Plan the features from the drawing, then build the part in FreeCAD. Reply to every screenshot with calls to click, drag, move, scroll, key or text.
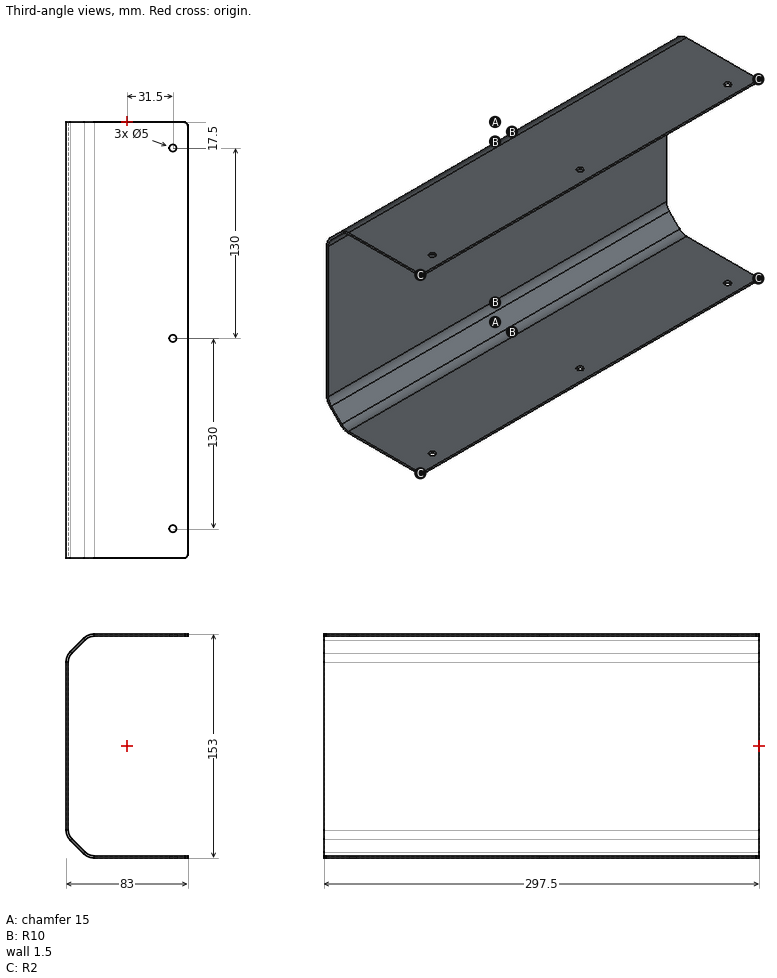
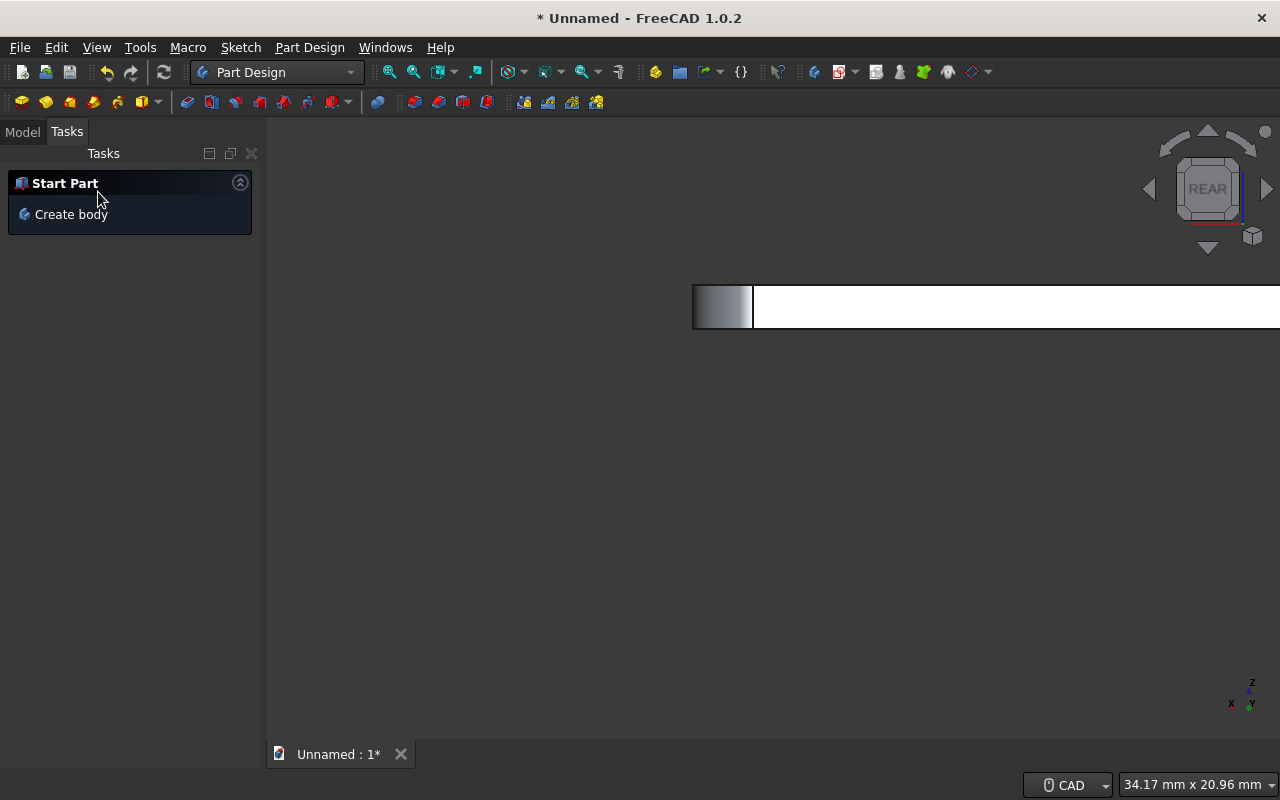
key(0)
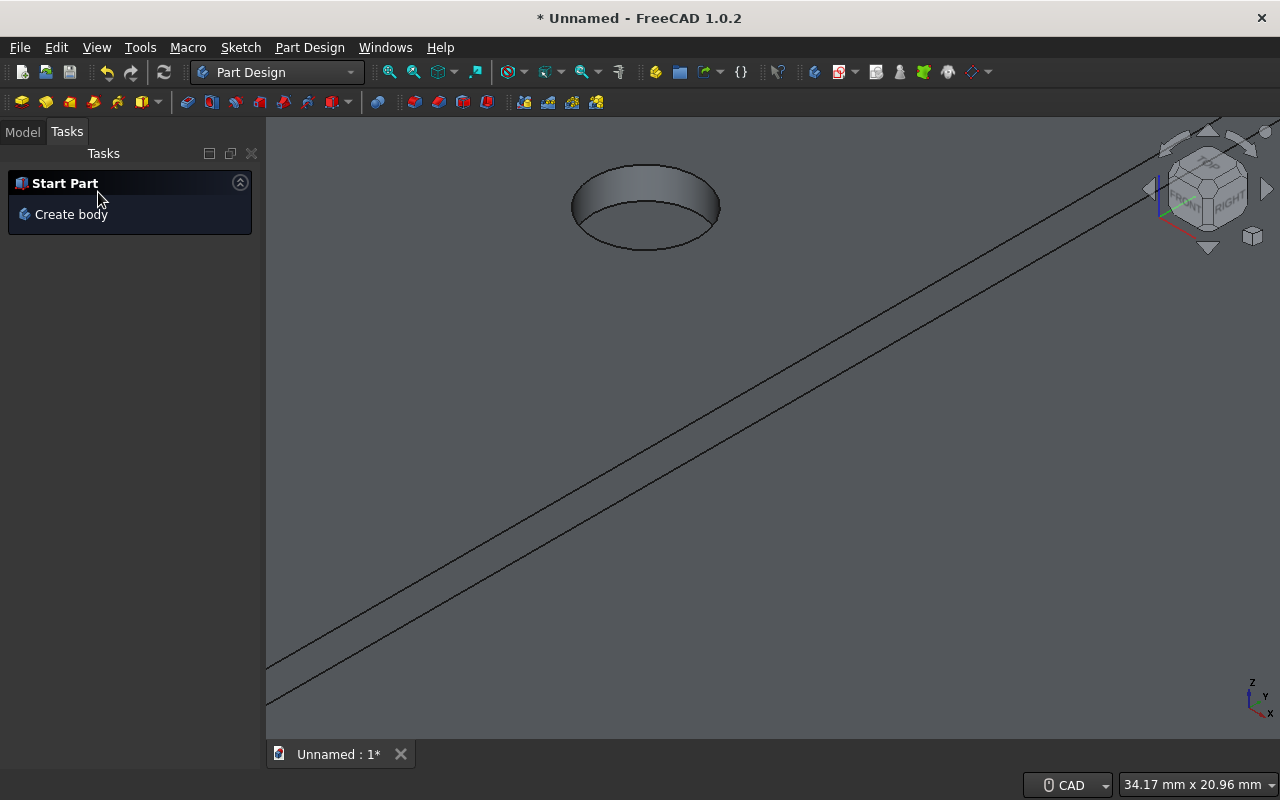
click(390, 72)